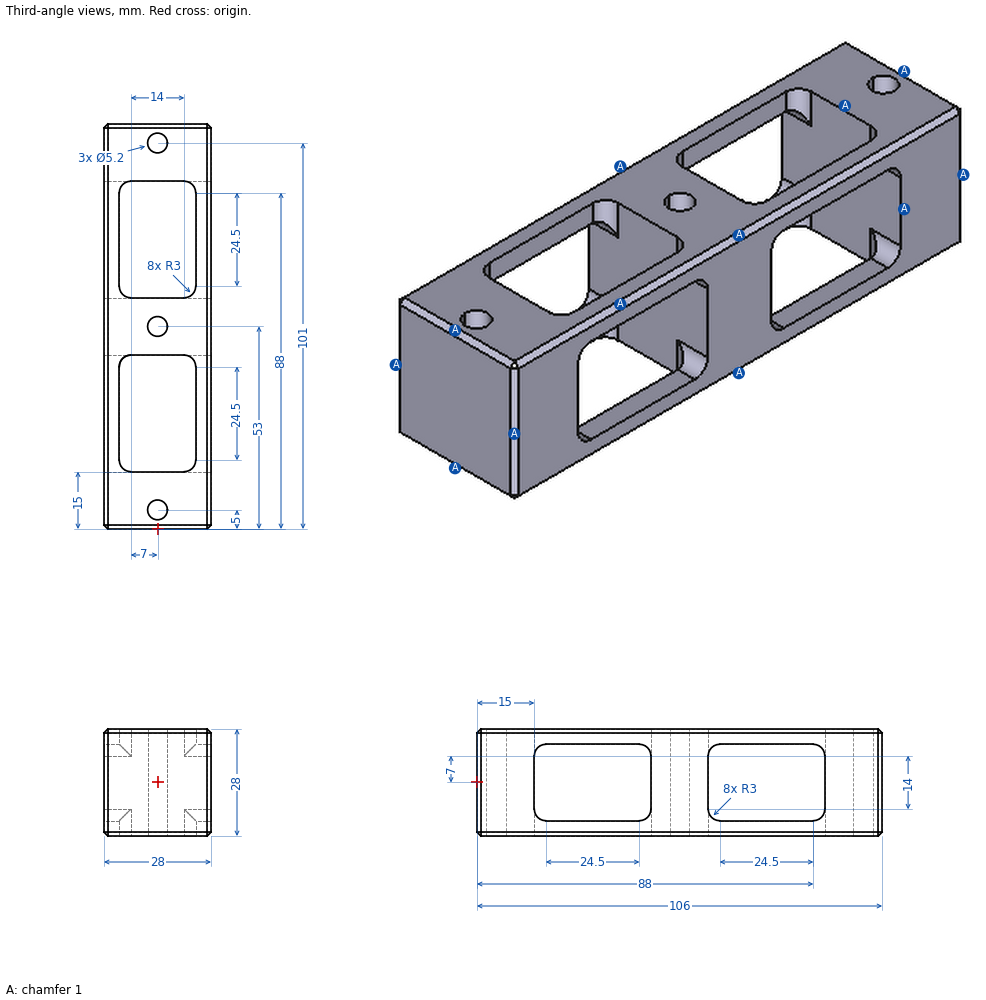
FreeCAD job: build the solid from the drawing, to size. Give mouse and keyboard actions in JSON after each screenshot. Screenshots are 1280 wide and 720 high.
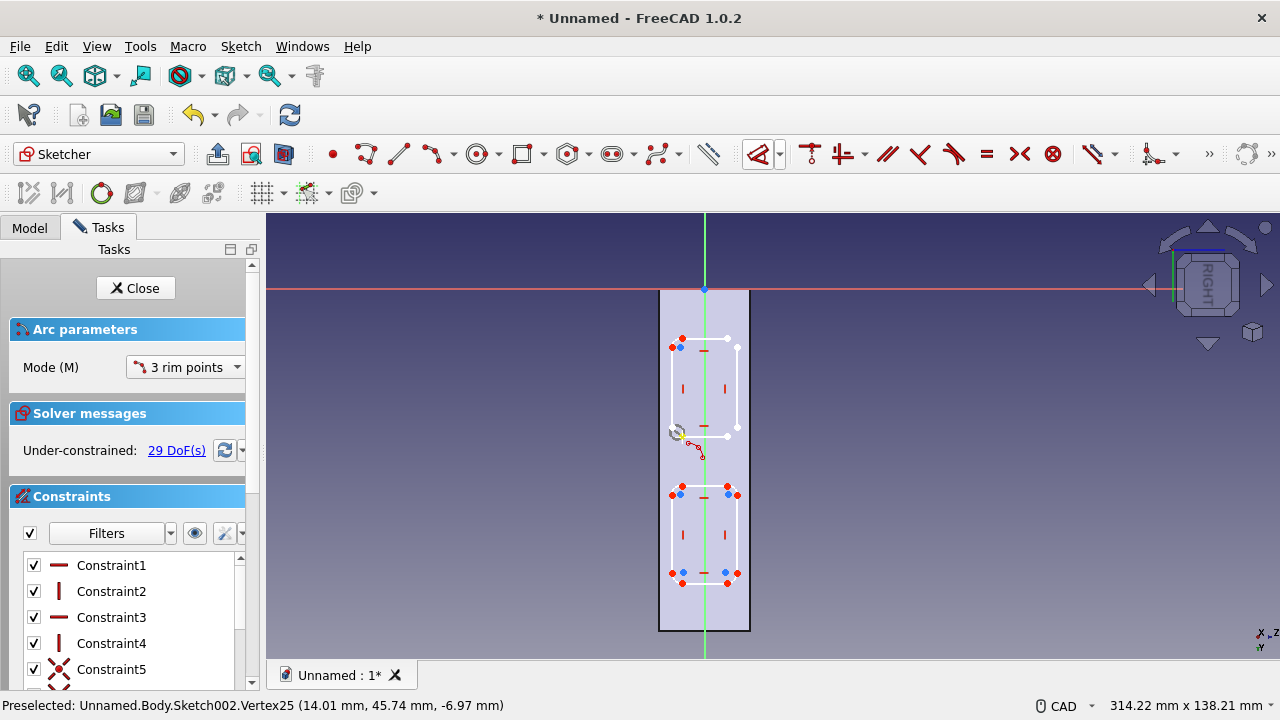
{"action": "scroll", "coordinate": [675, 433], "scroll_direction": "up", "scroll_amount": 9}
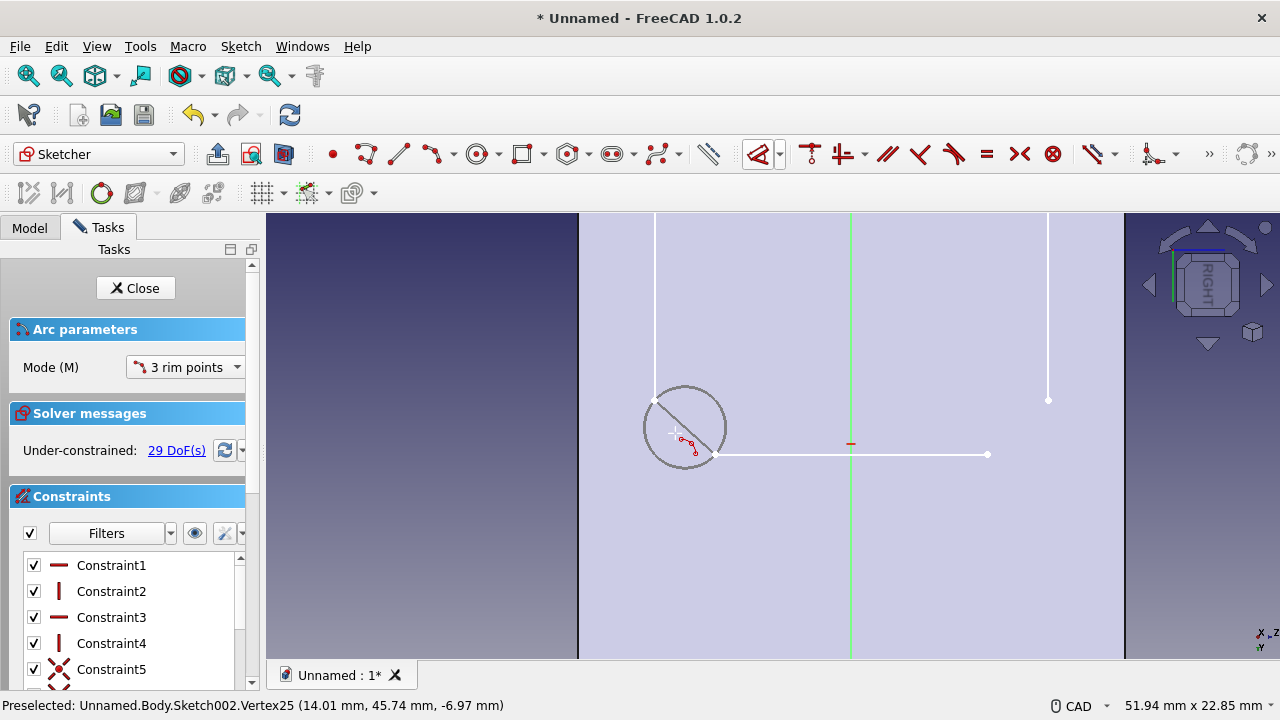
{"action": "left_click", "coordinate": [673, 433]}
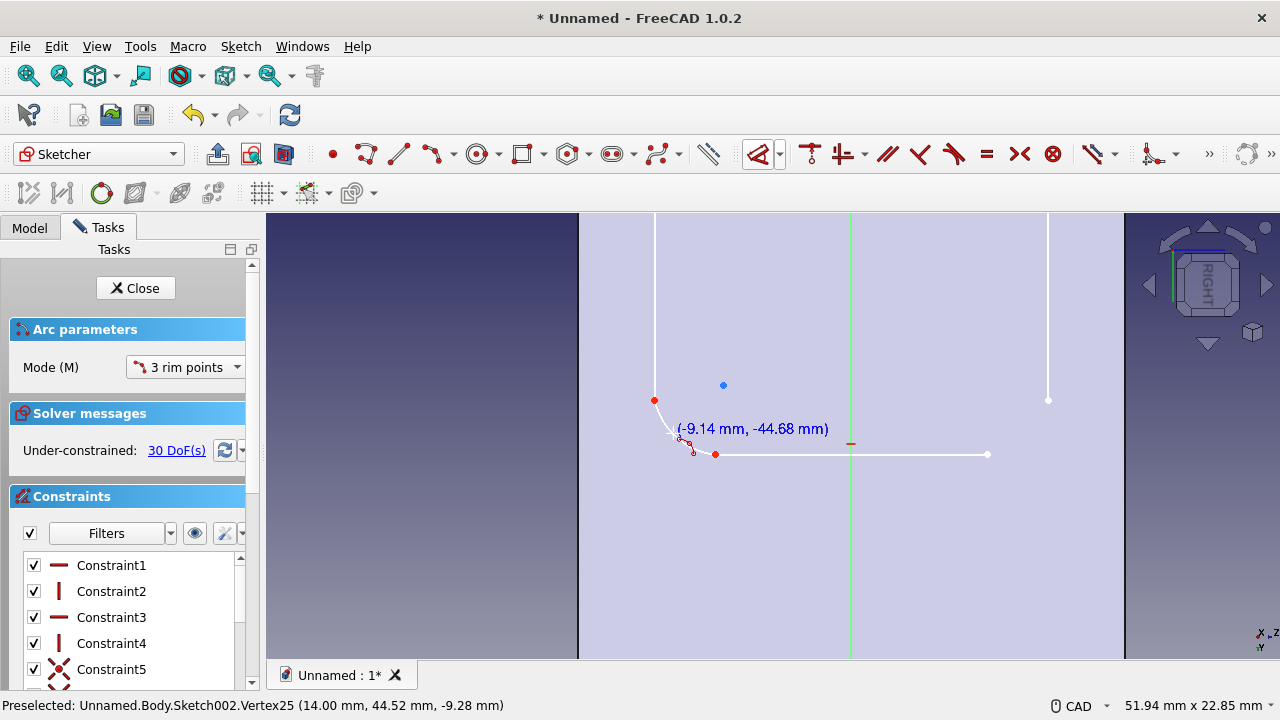
{"action": "scroll", "coordinate": [675, 433], "scroll_direction": "down", "scroll_amount": 9}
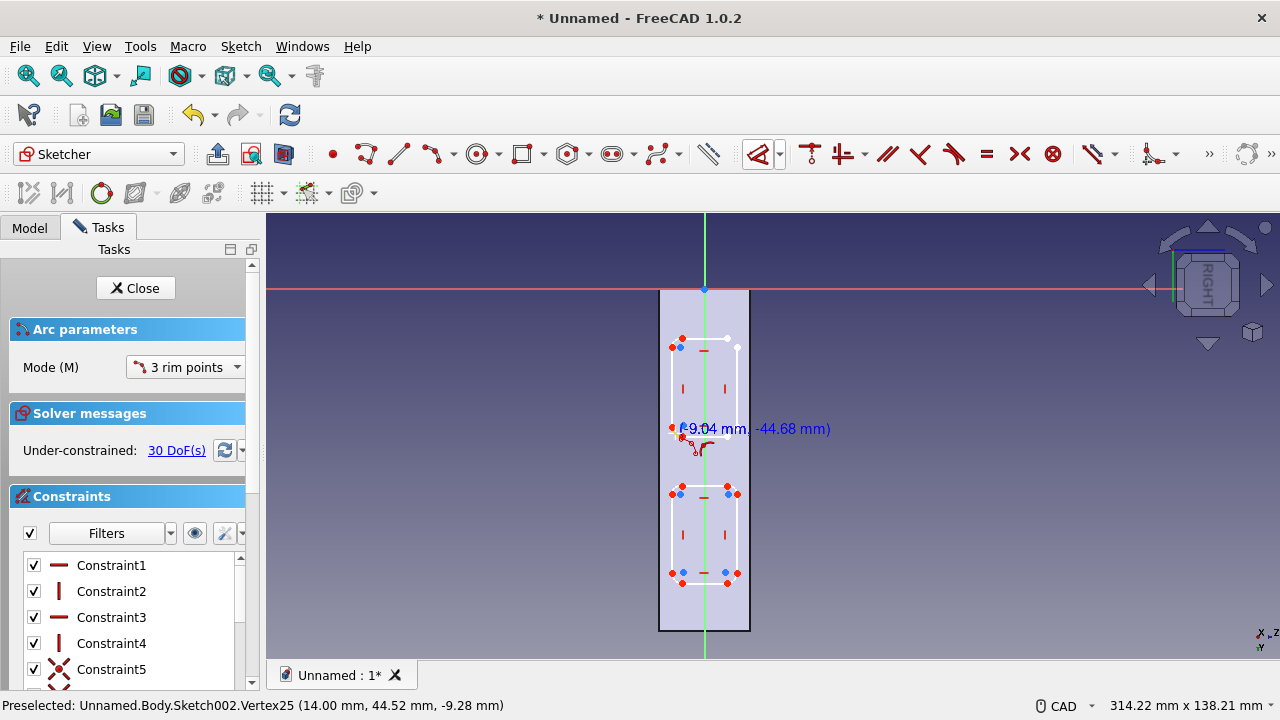
{"action": "left_click", "coordinate": [727, 437]}
{"action": "left_click", "coordinate": [737, 428]}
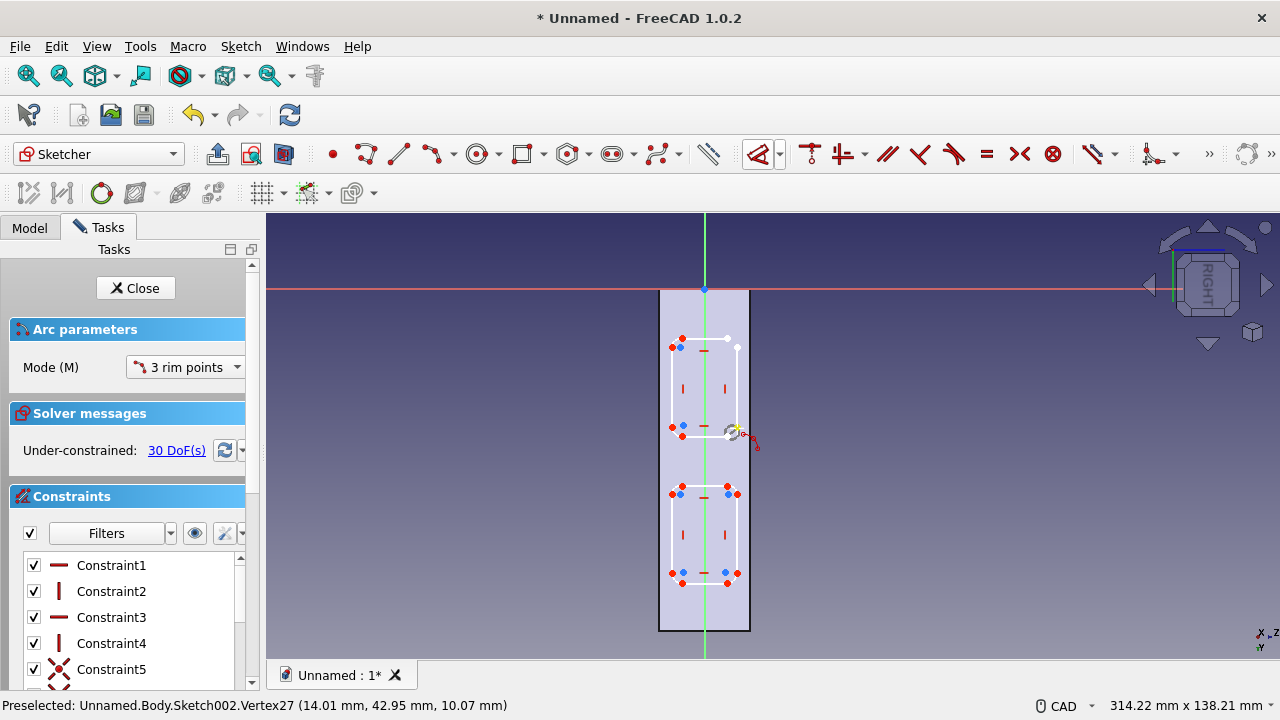
{"action": "scroll", "coordinate": [734, 433], "scroll_direction": "up", "scroll_amount": 9}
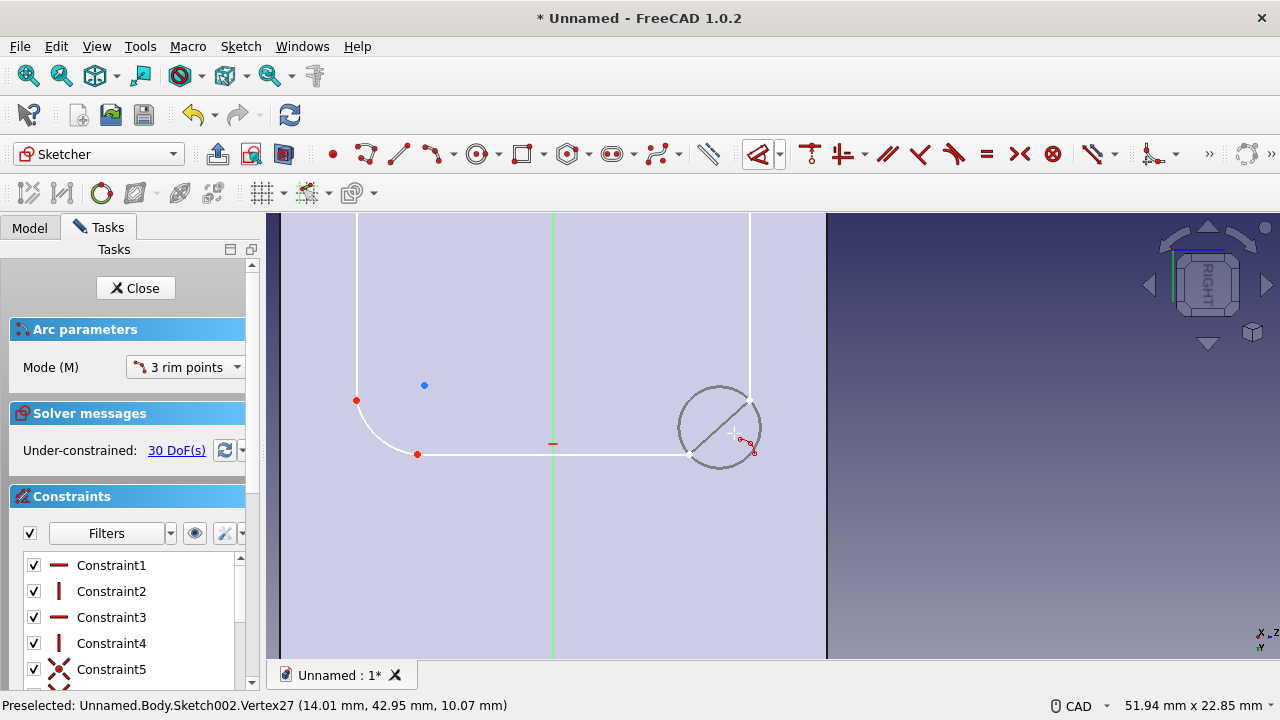
{"action": "left_click", "coordinate": [731, 433]}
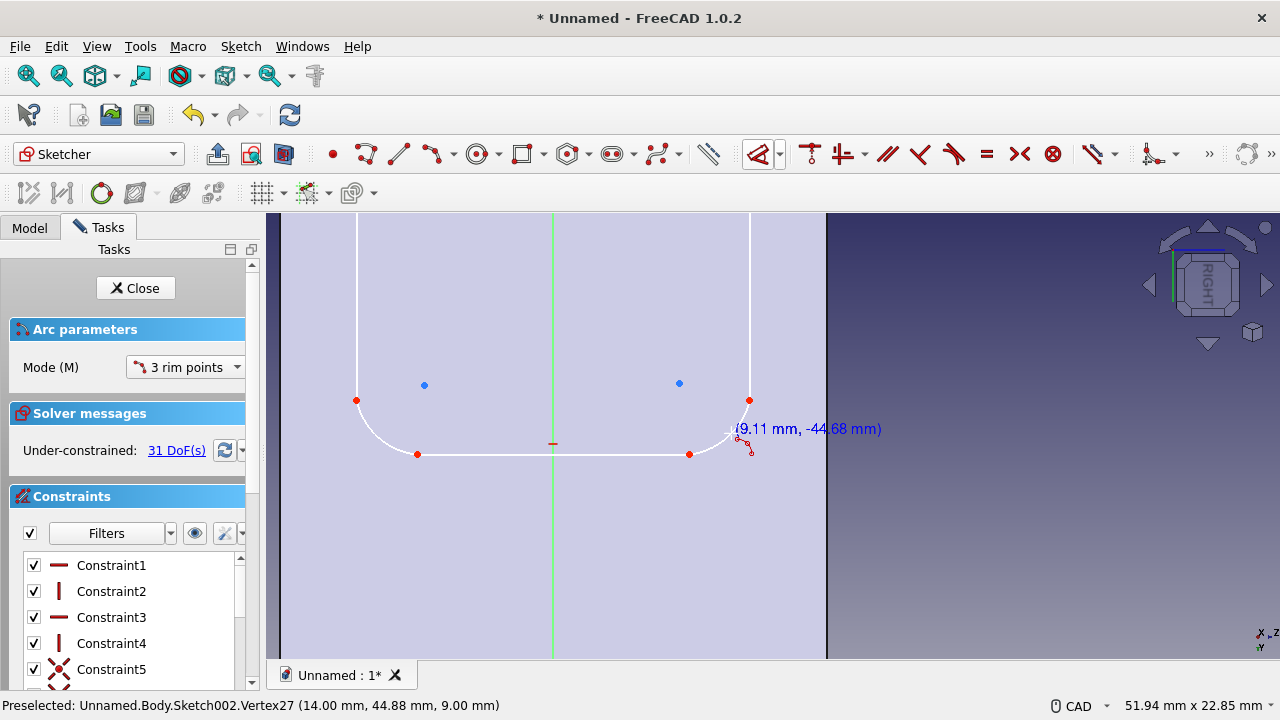
{"action": "scroll", "coordinate": [734, 433], "scroll_direction": "down", "scroll_amount": 9}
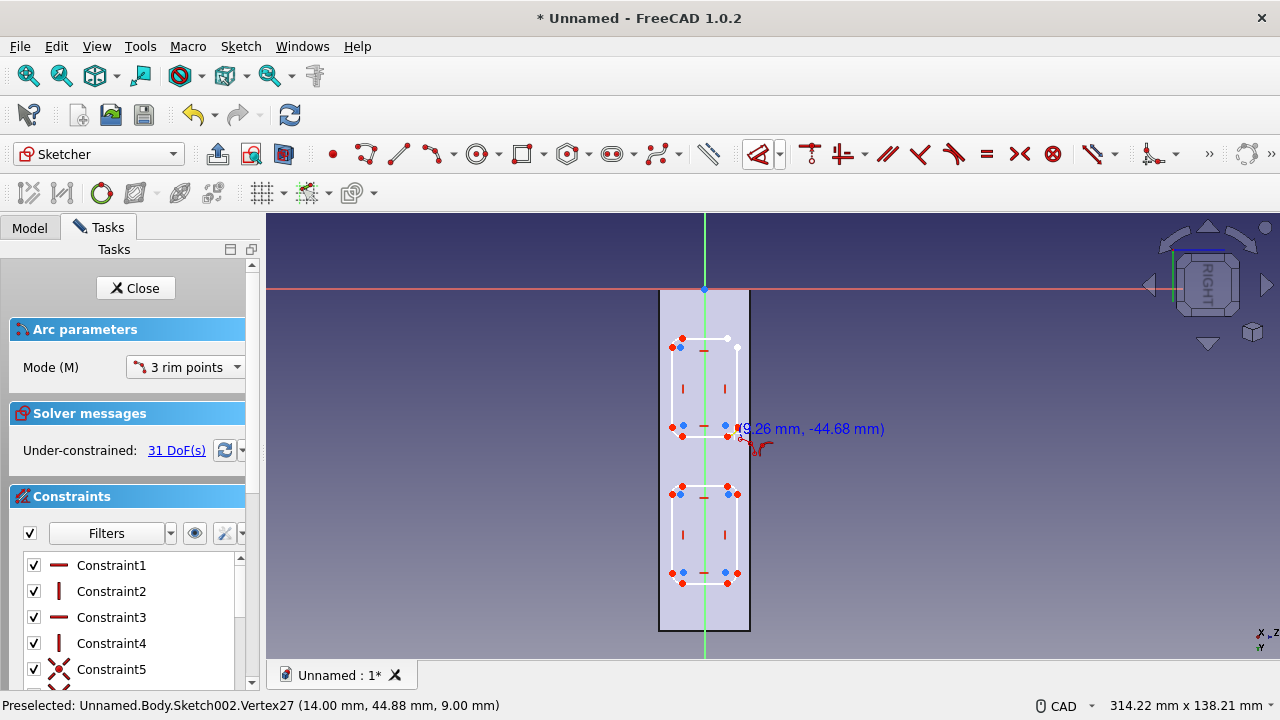
{"action": "left_click", "coordinate": [737, 348]}
{"action": "left_click", "coordinate": [727, 339]}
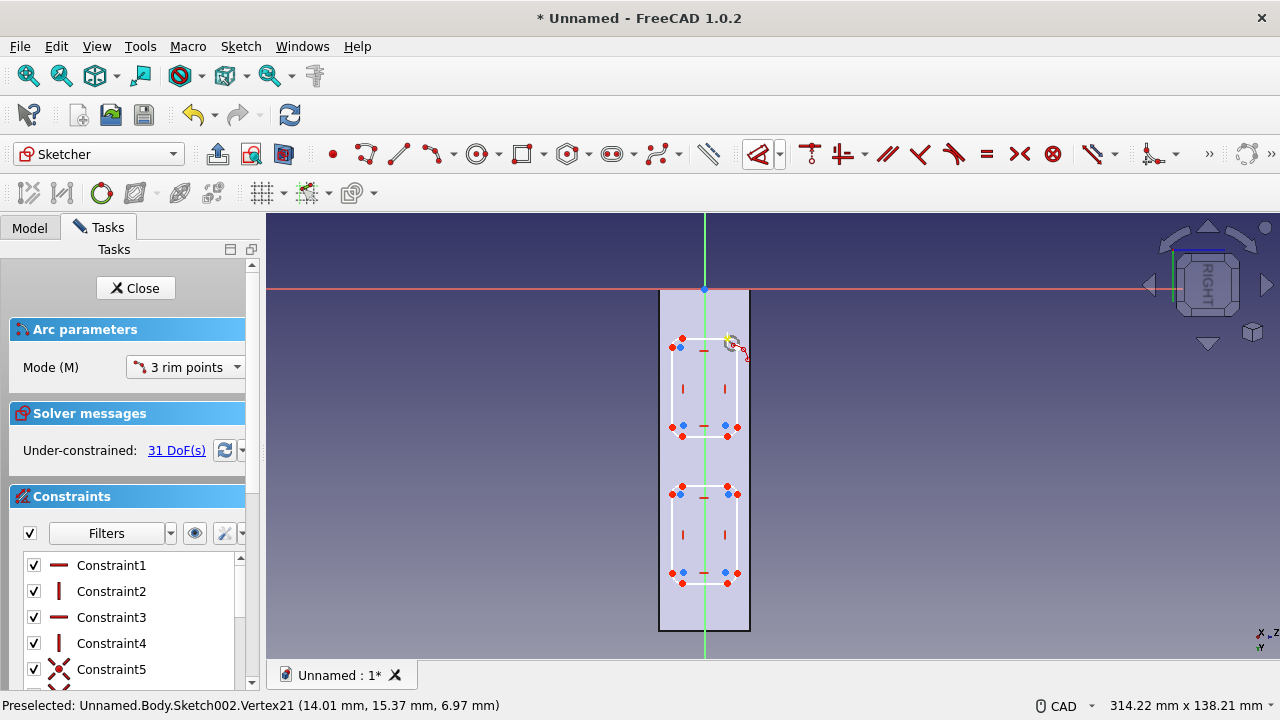
{"action": "scroll", "coordinate": [734, 341], "scroll_direction": "up", "scroll_amount": 9}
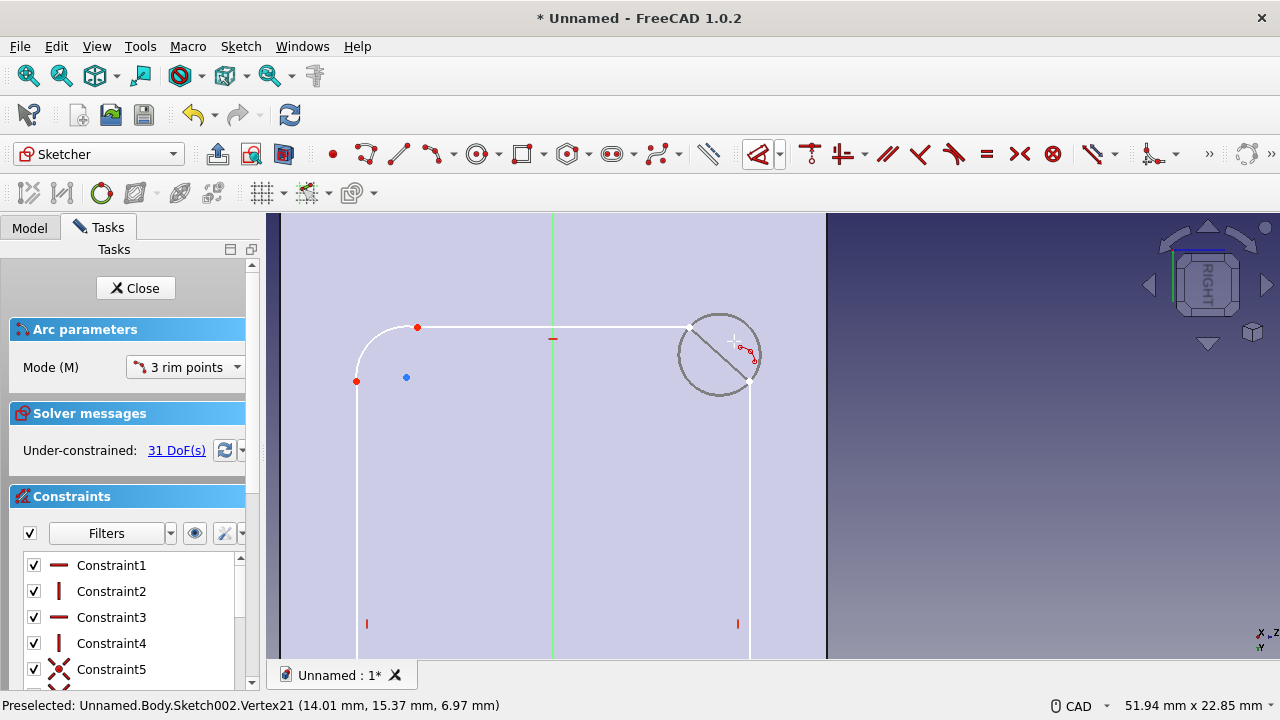
{"action": "left_click", "coordinate": [731, 337]}
{"action": "key", "text": "Escape"}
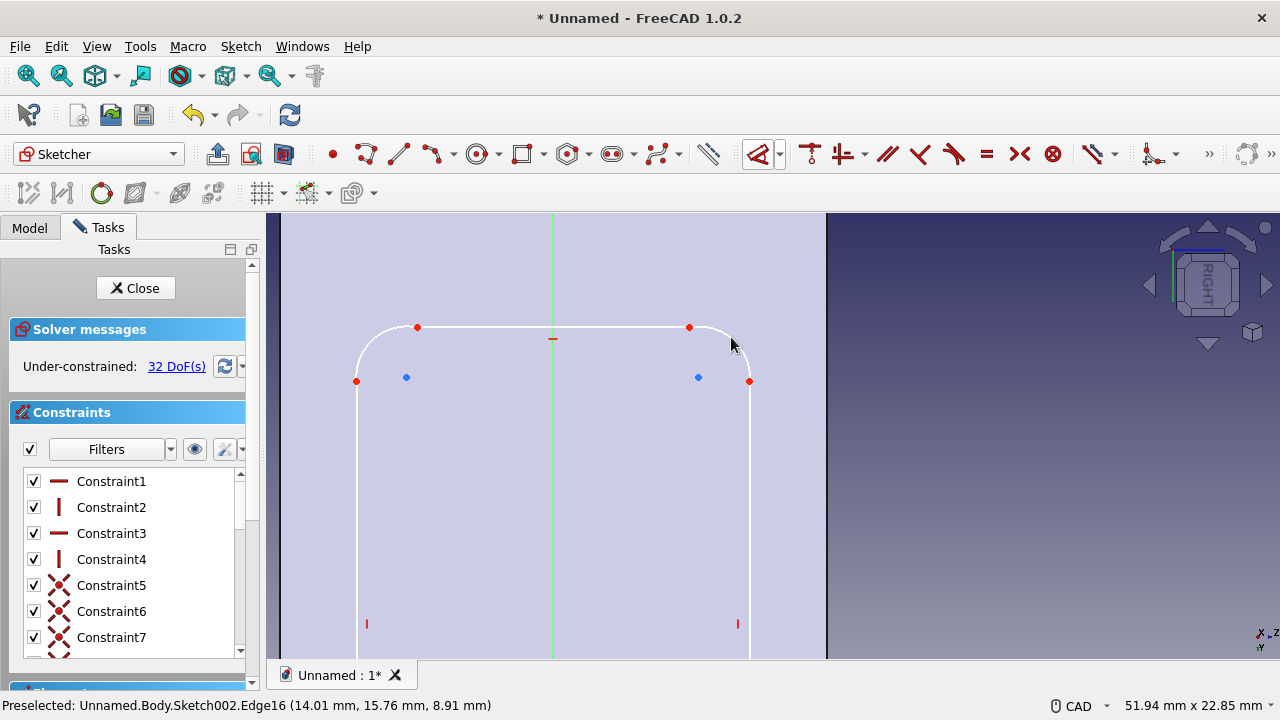
{"action": "scroll", "coordinate": [734, 341], "scroll_direction": "down", "scroll_amount": 9}